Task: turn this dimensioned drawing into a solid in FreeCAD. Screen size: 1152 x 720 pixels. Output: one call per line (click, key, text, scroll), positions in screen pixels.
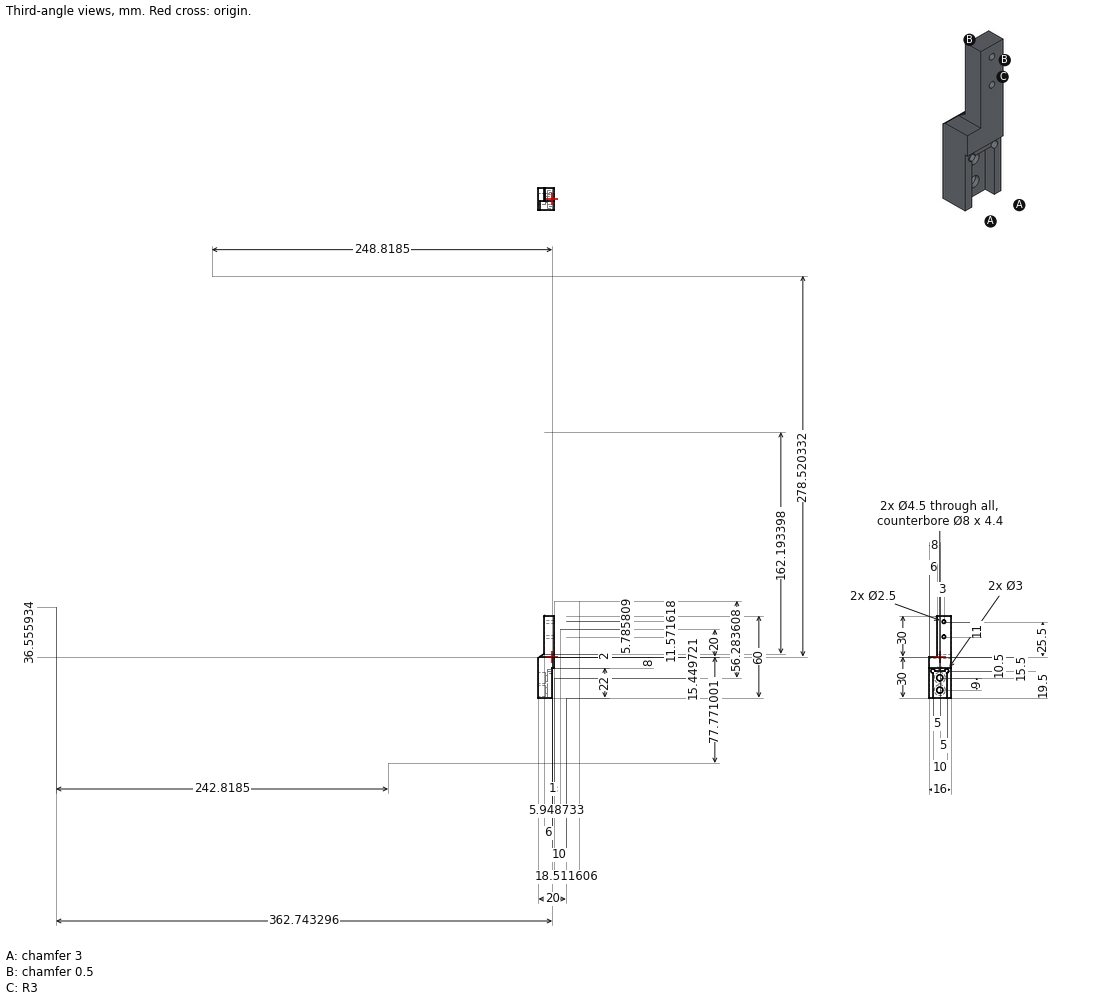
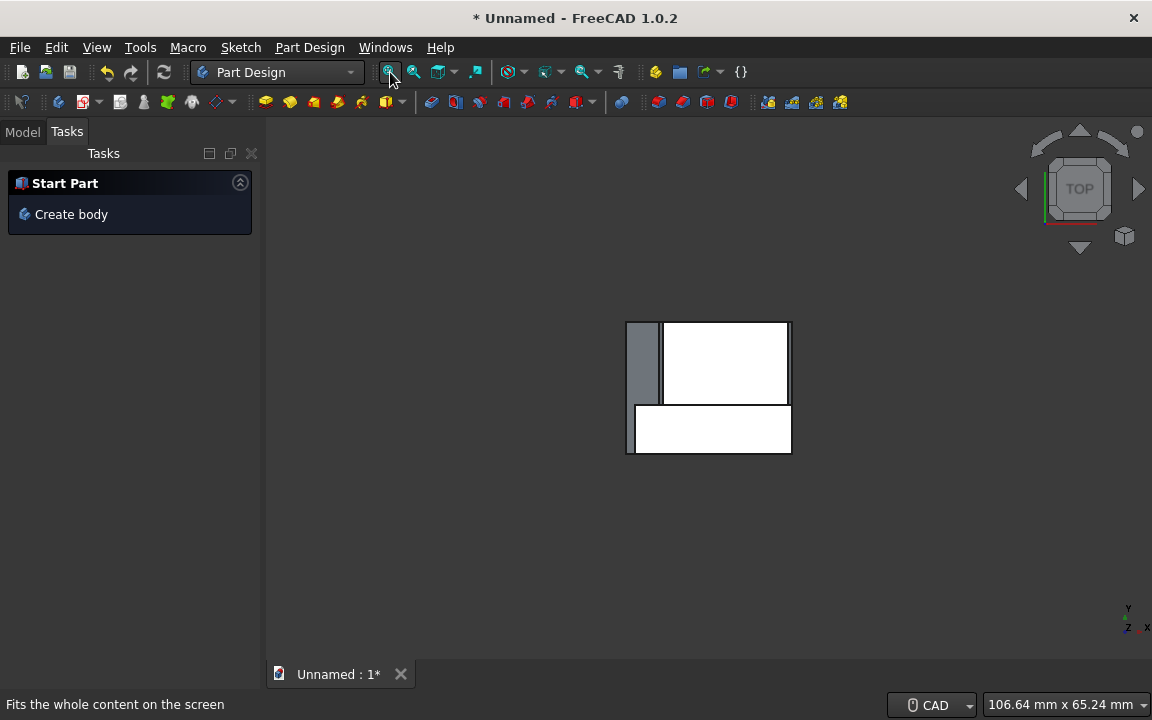
key(0)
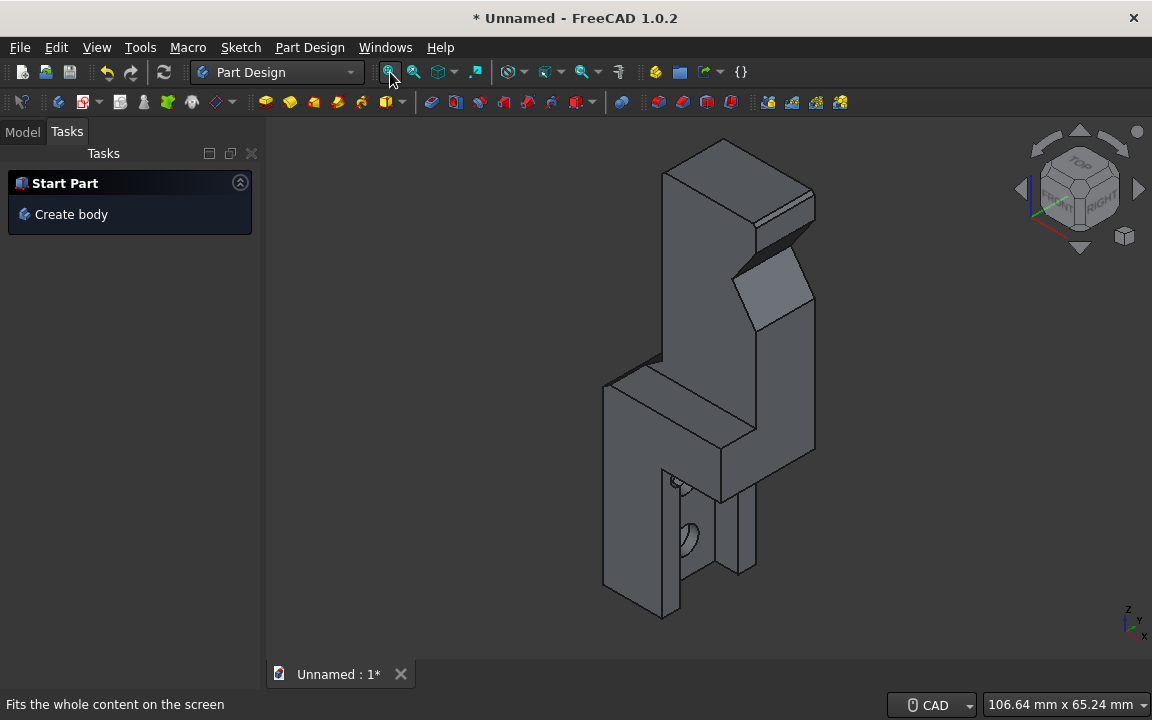
key(1)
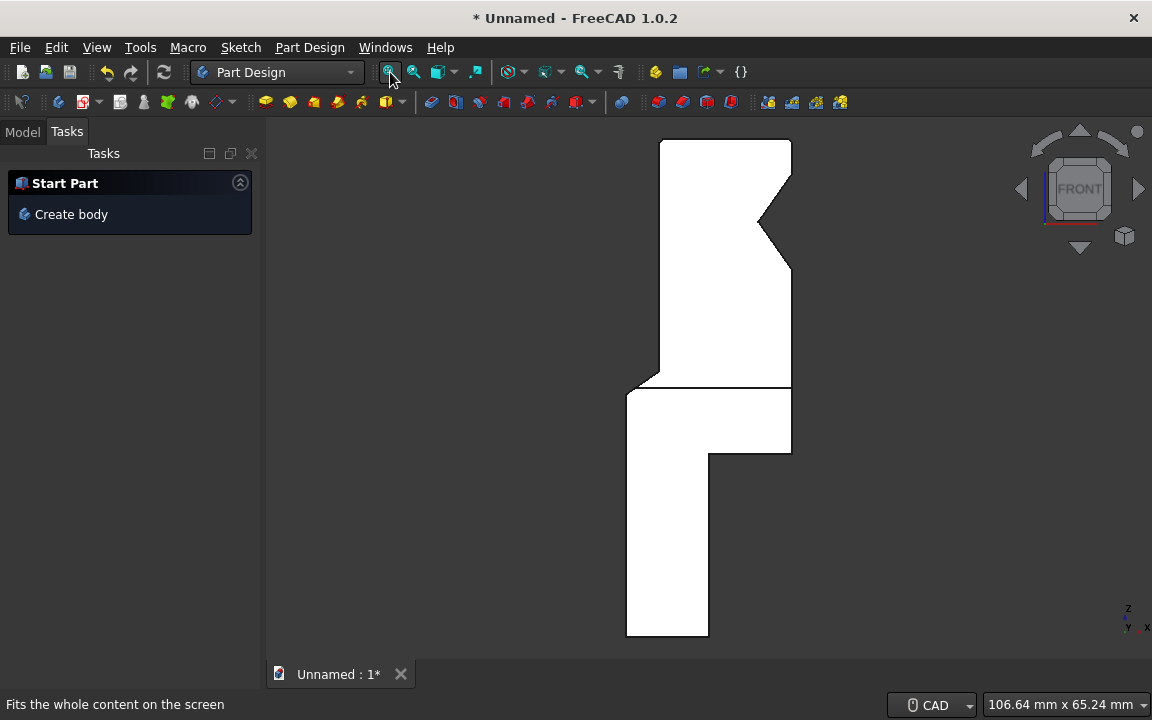
key(3)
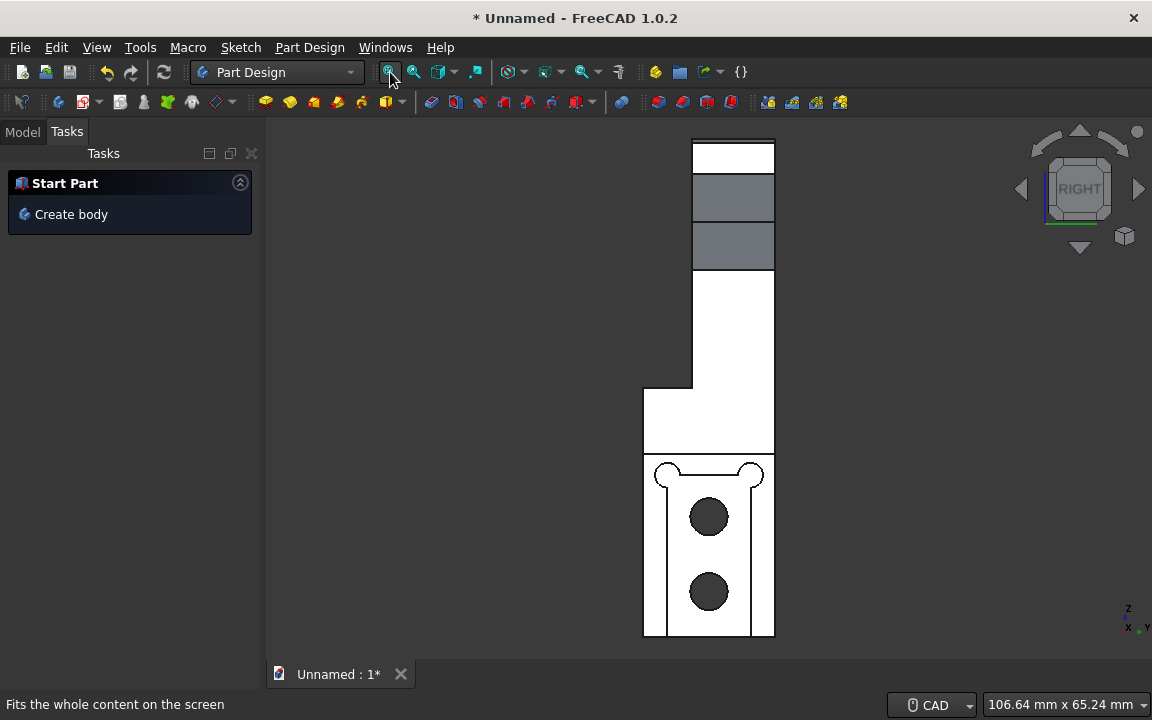
key(5)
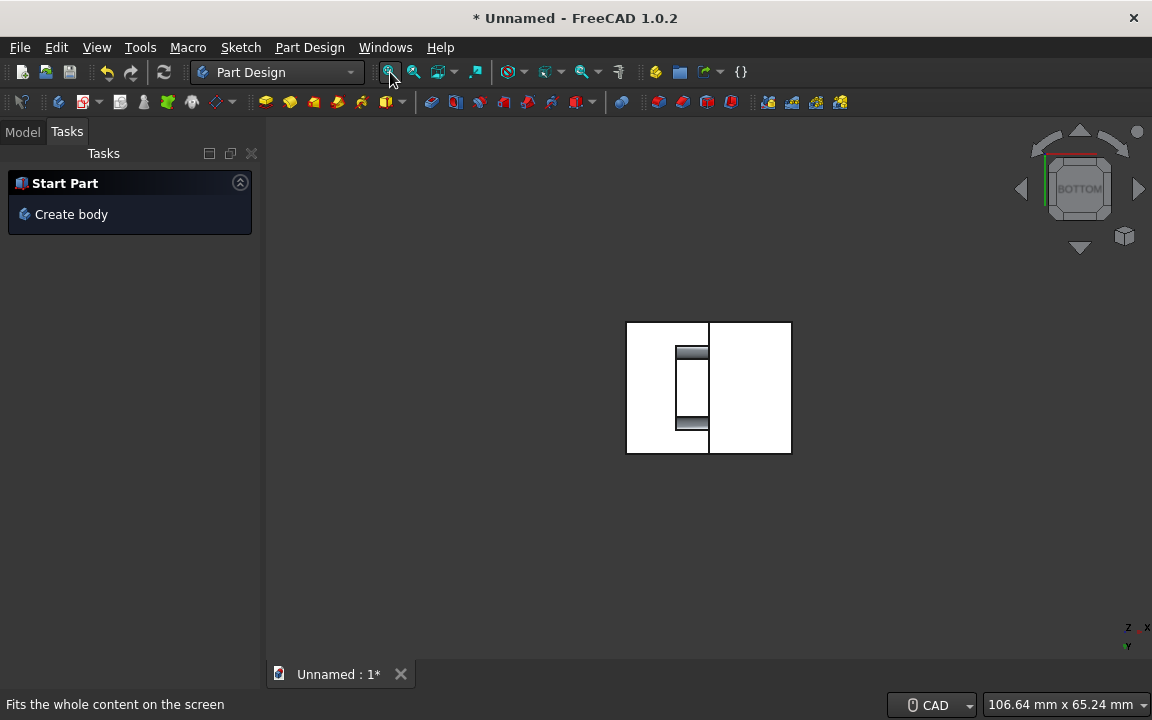
key(v)
key(f)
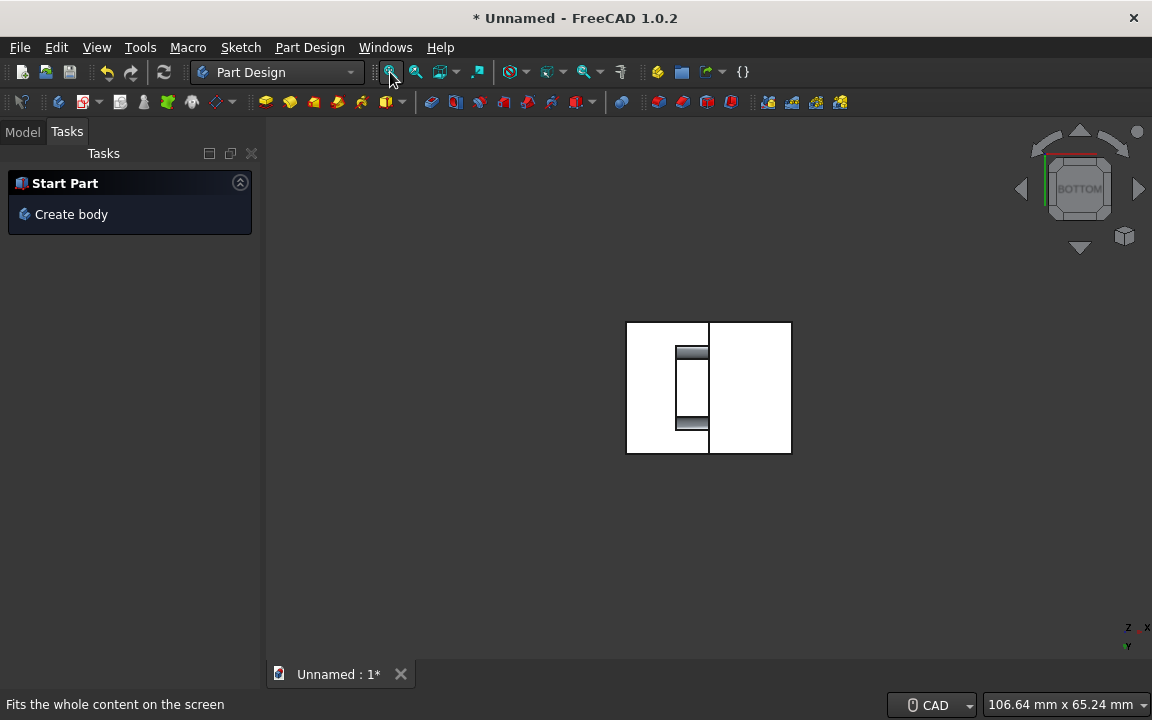
key(4)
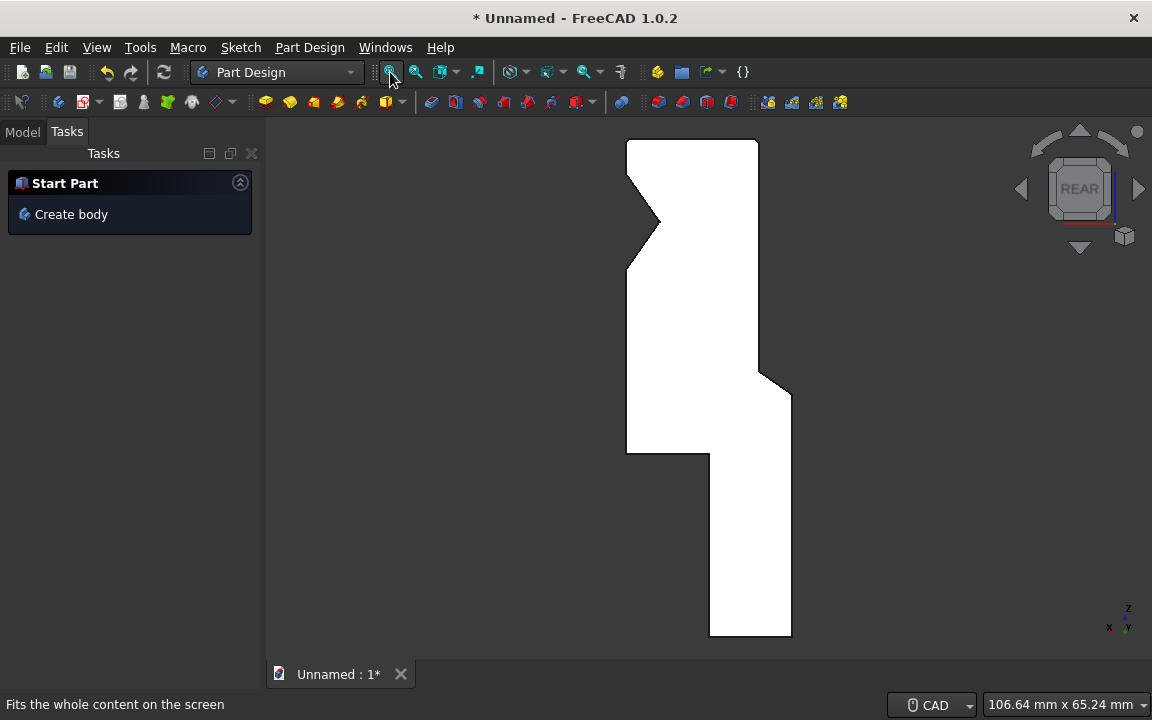
key(6)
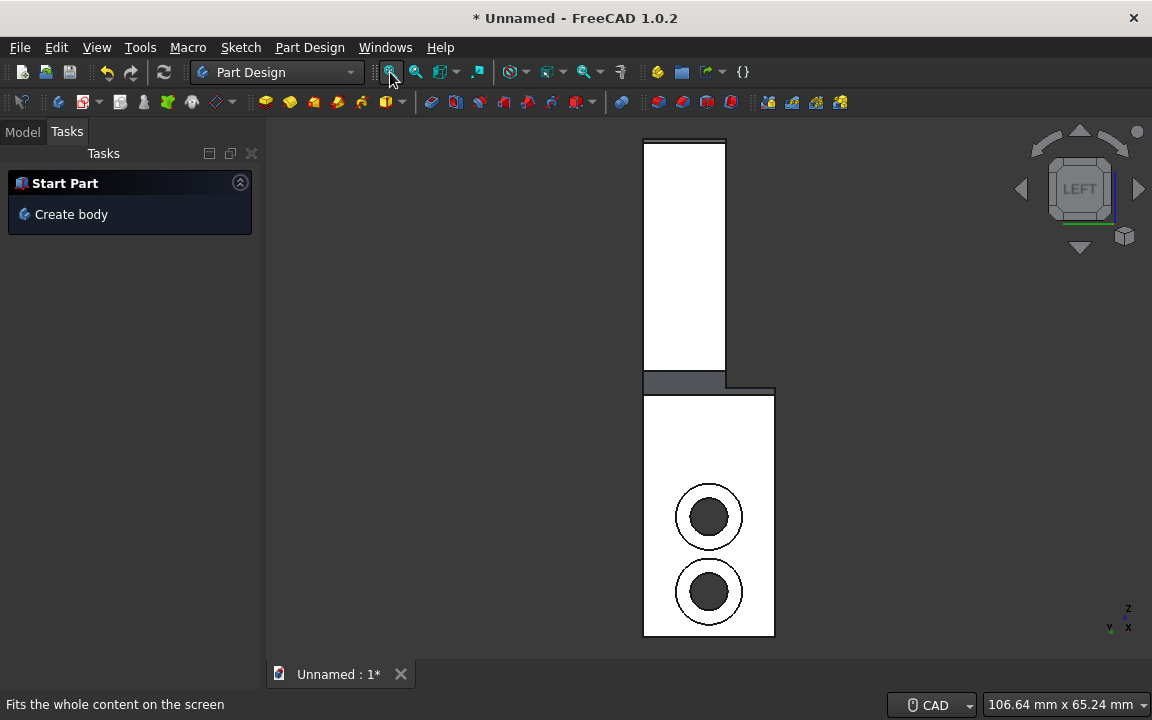
key(v)
key(3)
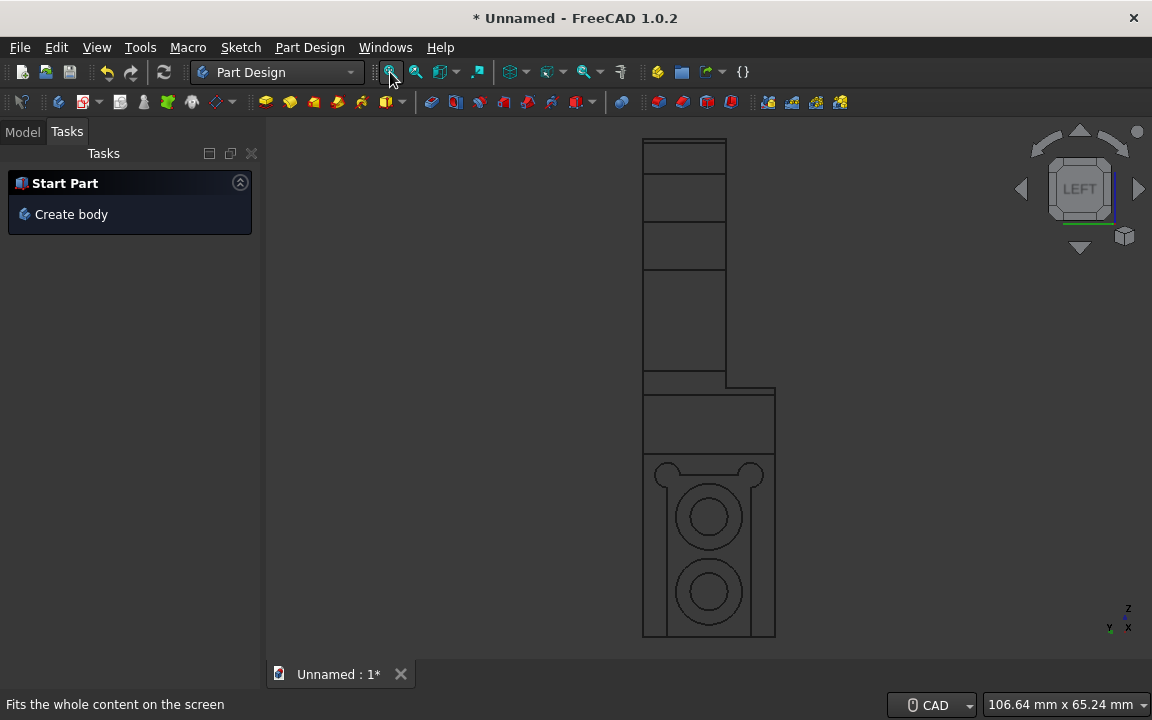
key(0)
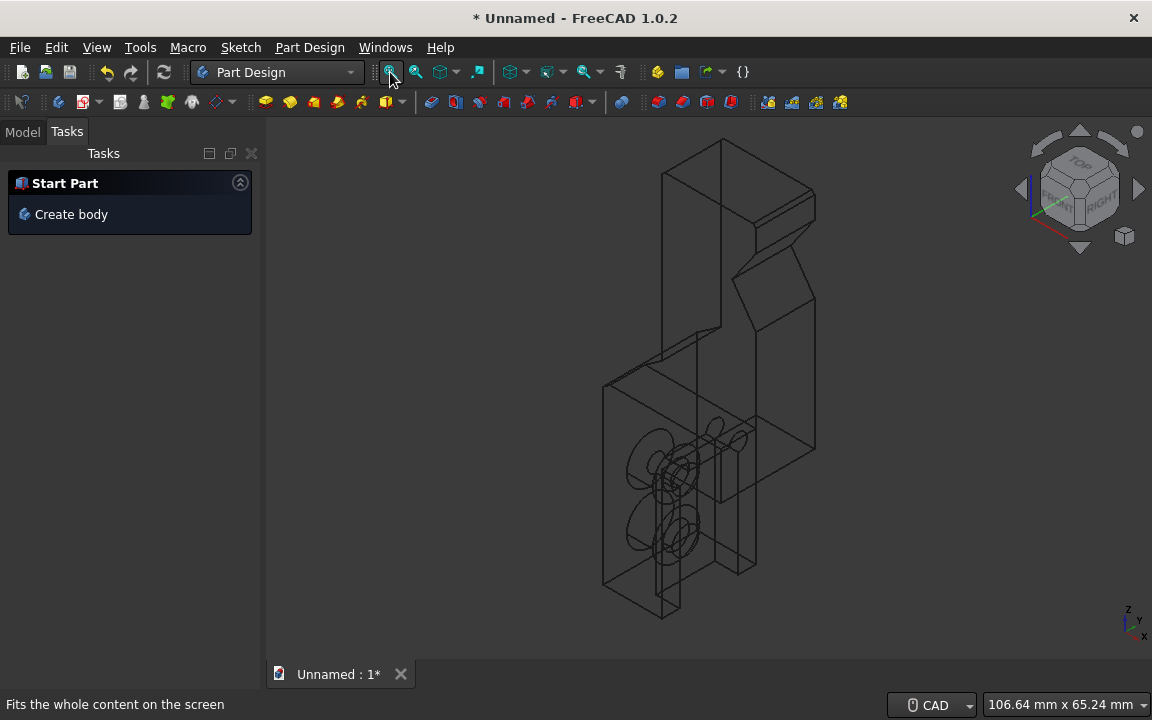
click(762, 261)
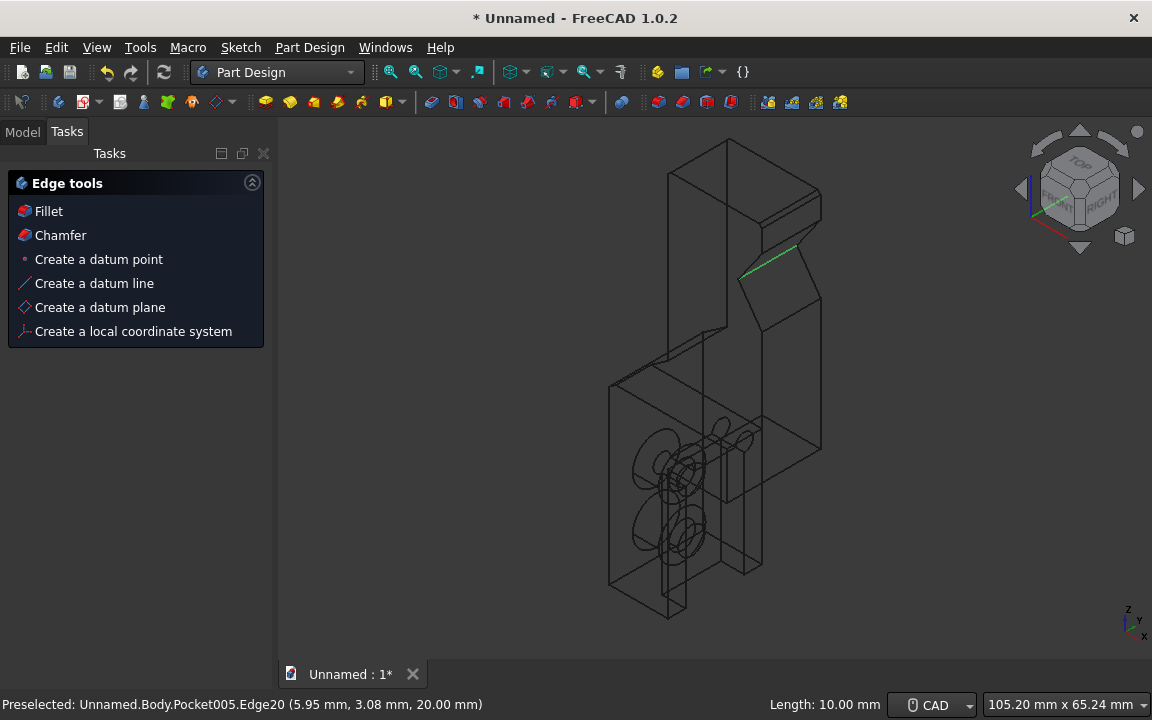
key(v)
key(1)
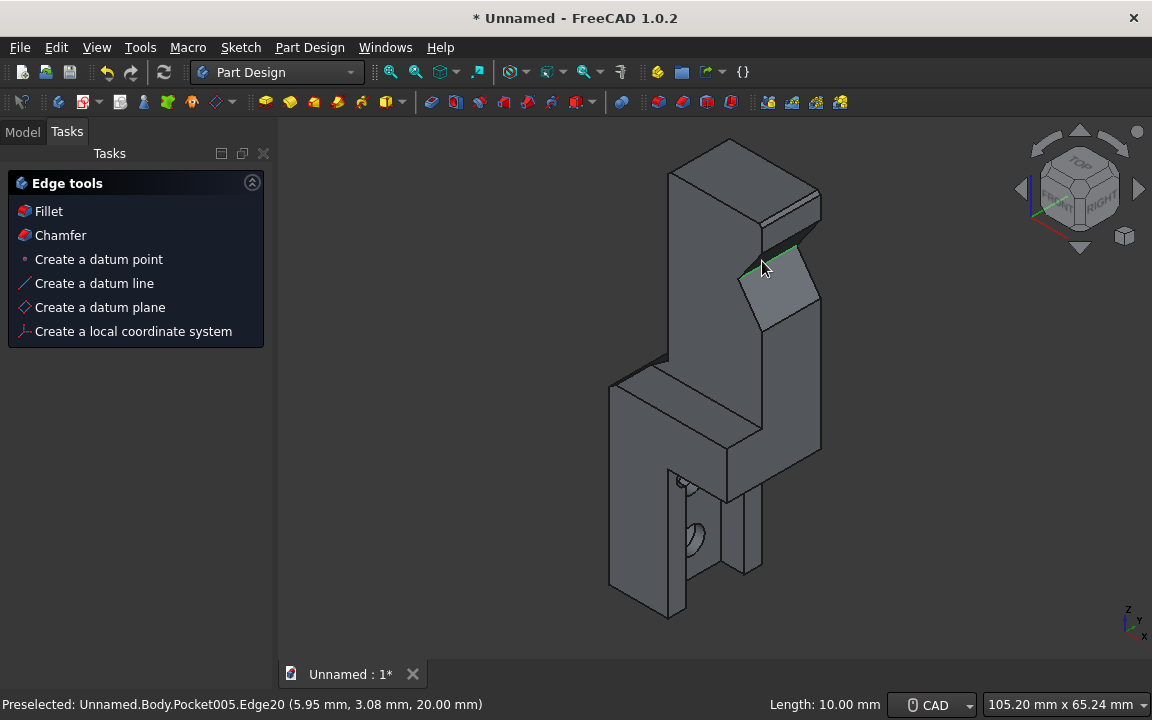
click(660, 102)